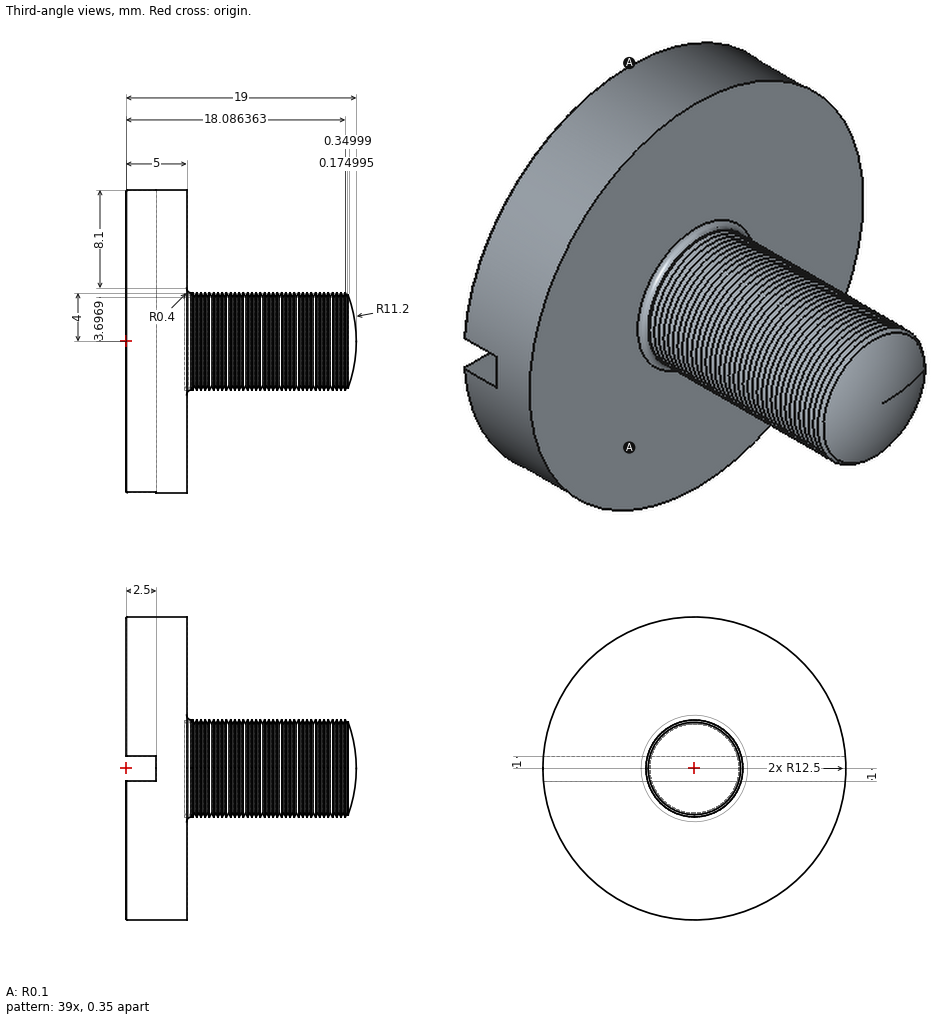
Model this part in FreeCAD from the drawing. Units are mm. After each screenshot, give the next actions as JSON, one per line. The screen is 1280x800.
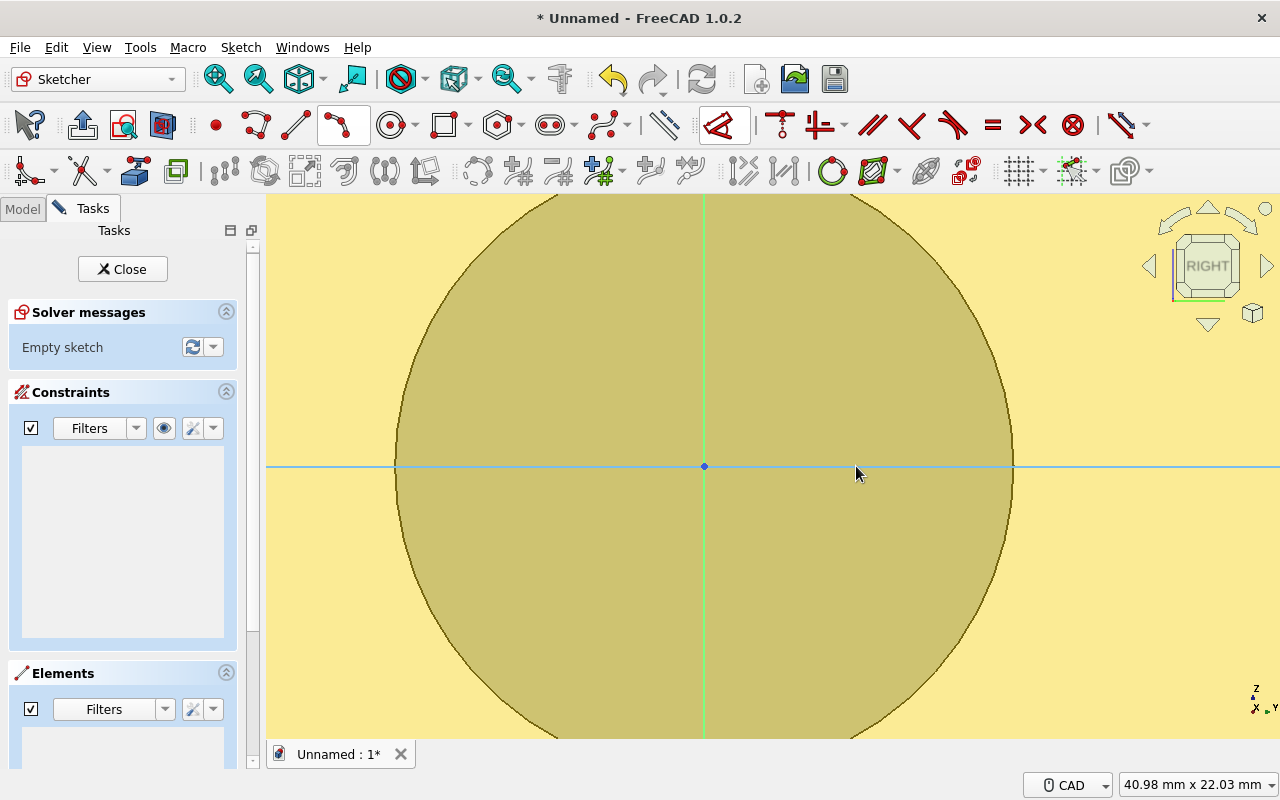
{"action": "left_click", "coordinate": [296, 126]}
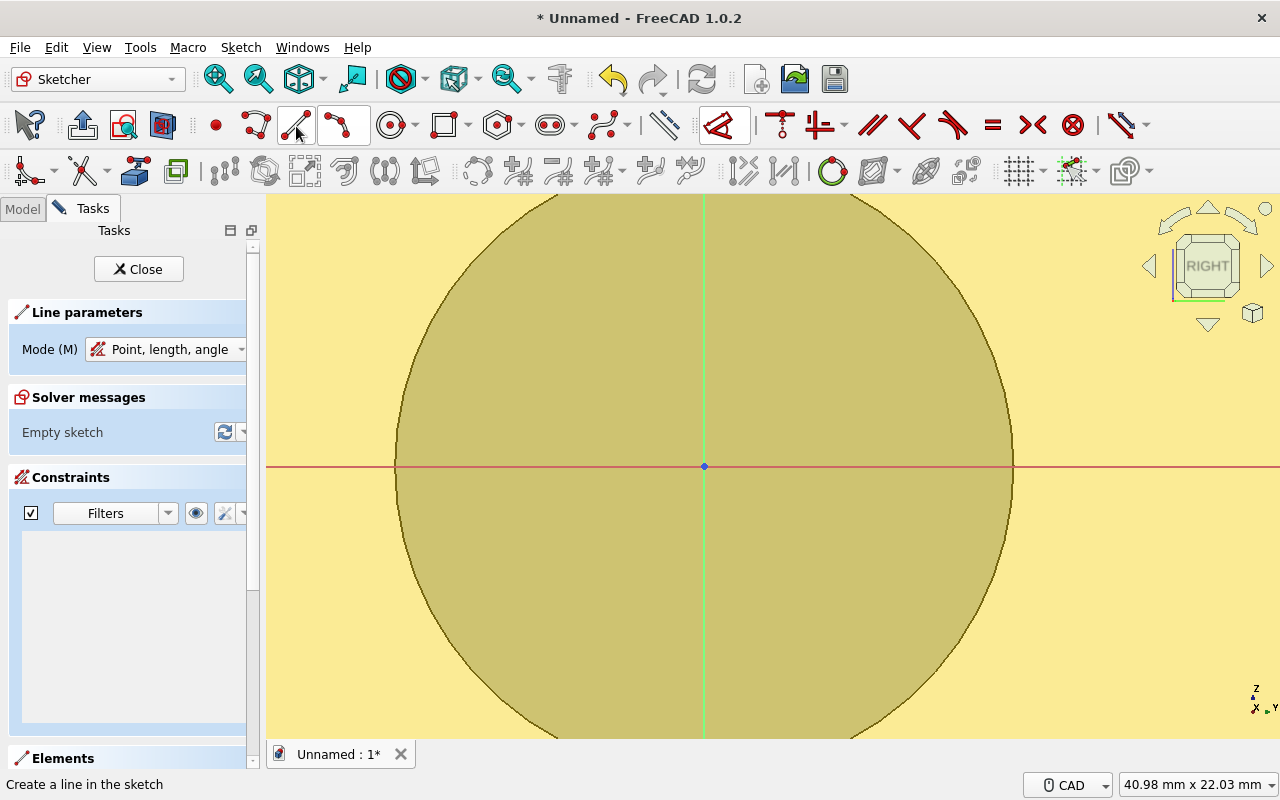
{"action": "left_click", "coordinate": [396, 442]}
{"action": "left_click", "coordinate": [1013, 442]}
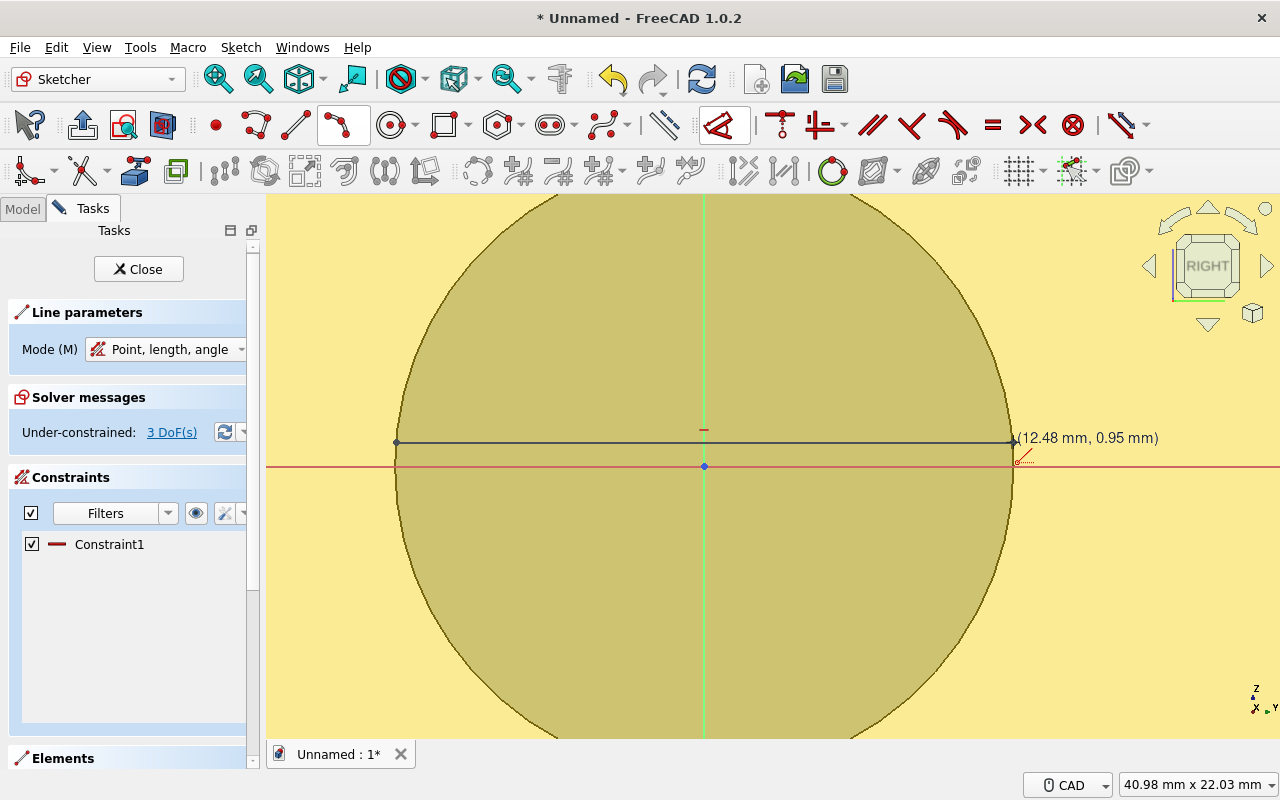
{"action": "left_click", "coordinate": [1013, 491]}
{"action": "left_click", "coordinate": [396, 491]}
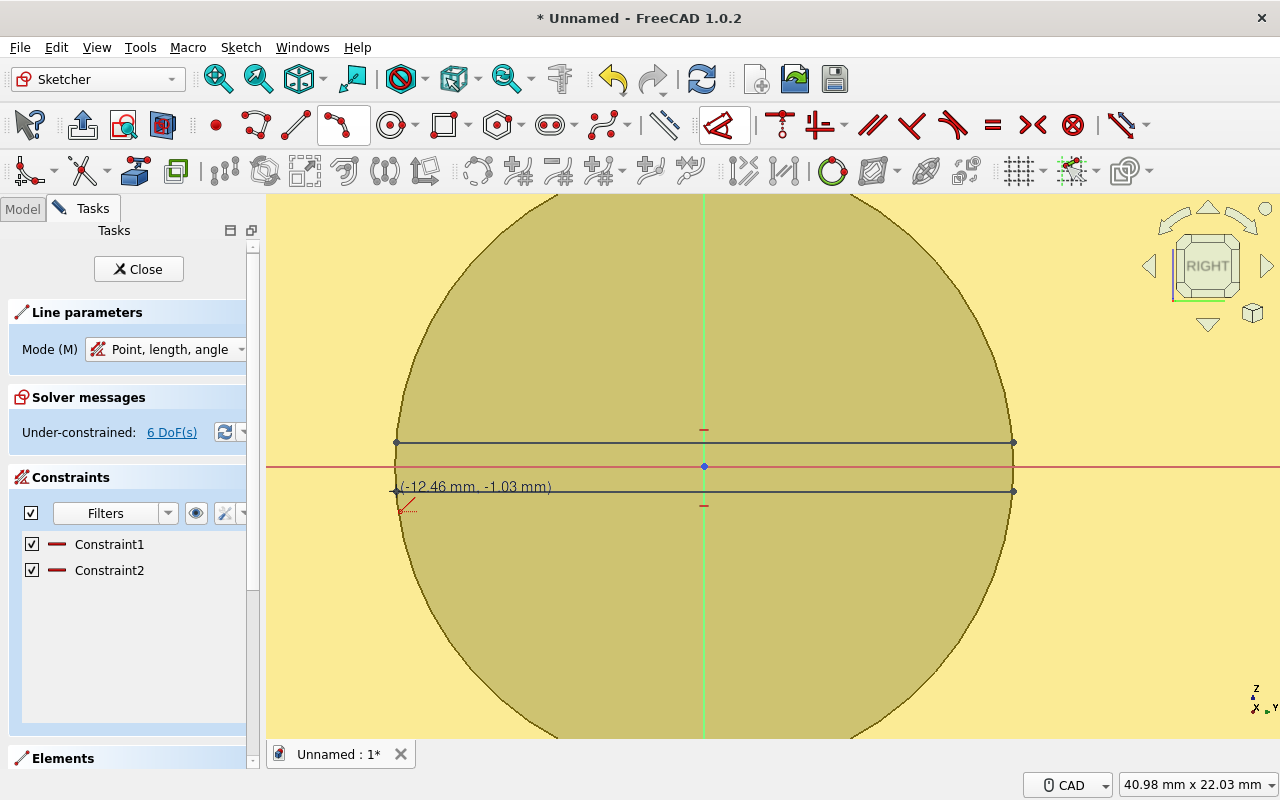
{"action": "left_click", "coordinate": [338, 126]}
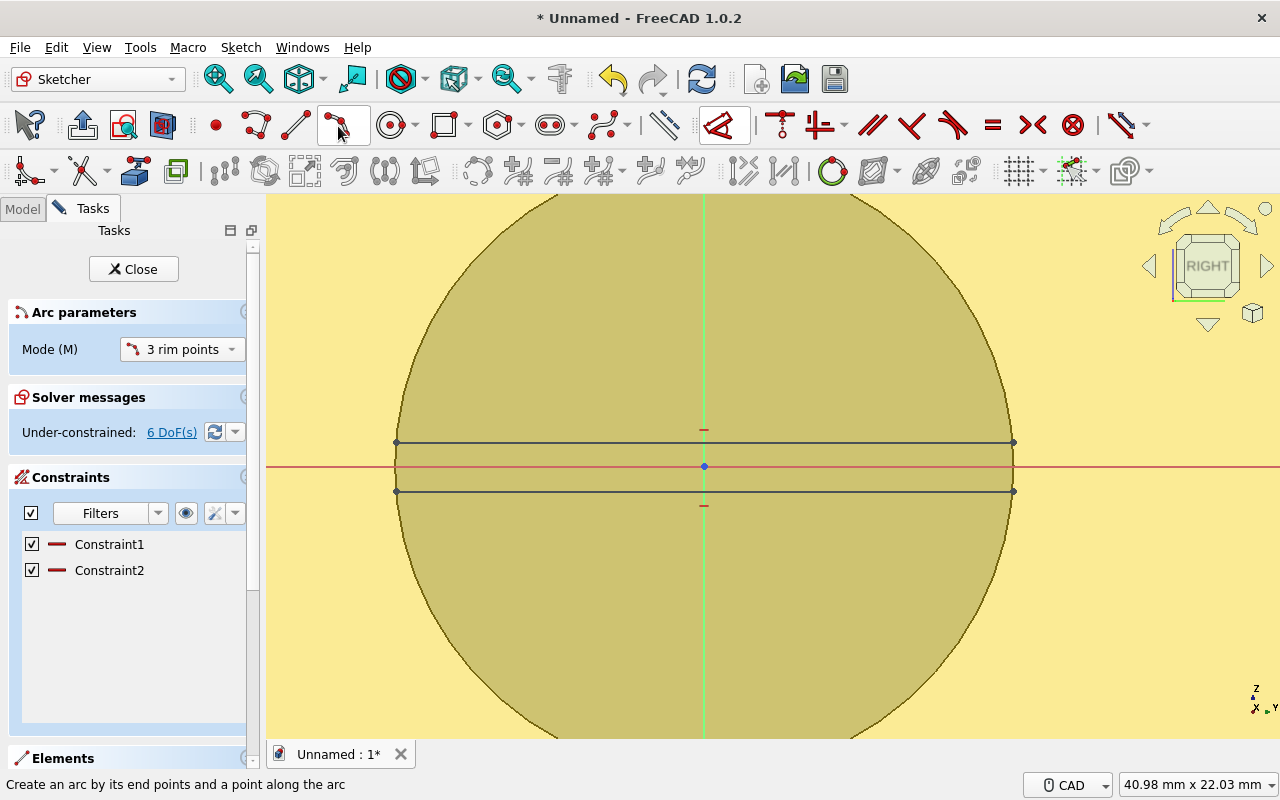
{"action": "left_click", "coordinate": [1013, 443]}
{"action": "left_click", "coordinate": [1013, 492]}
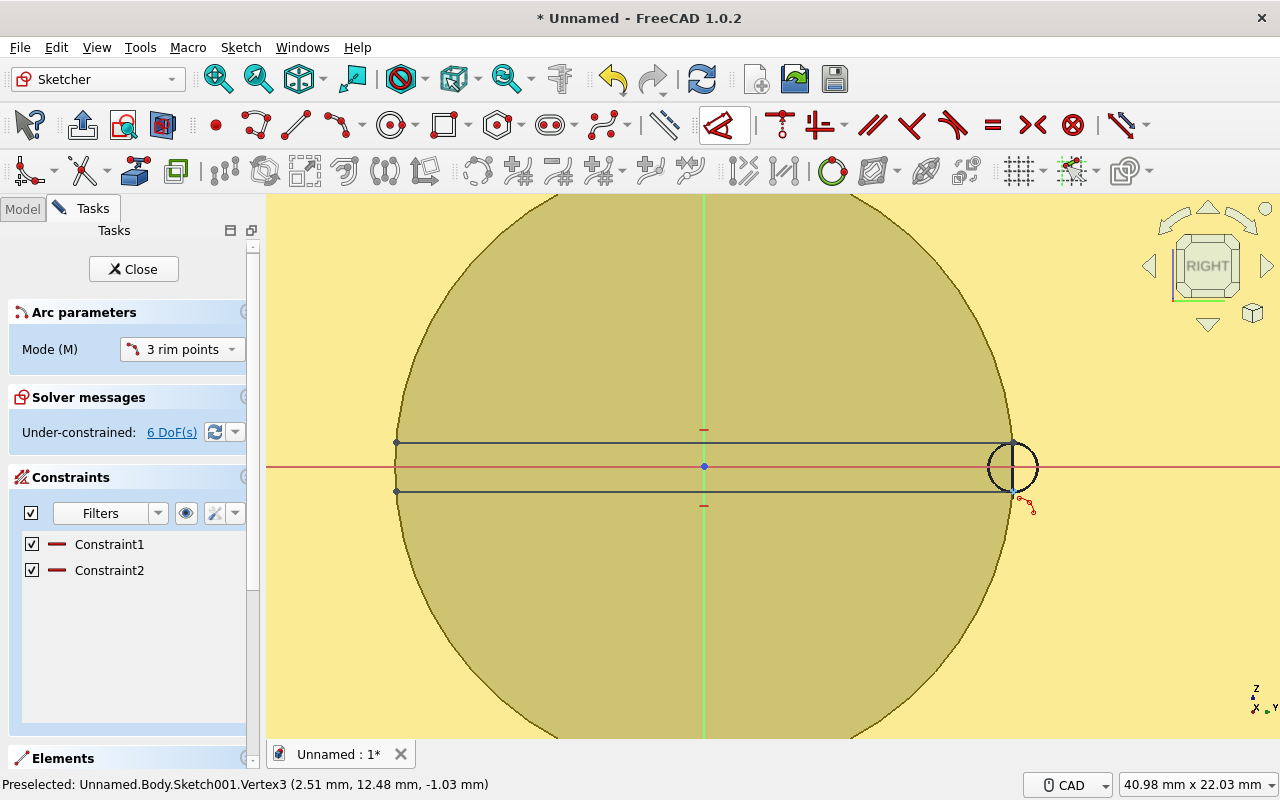
{"action": "scroll", "coordinate": [1014, 471], "scroll_direction": "up", "scroll_amount": 15}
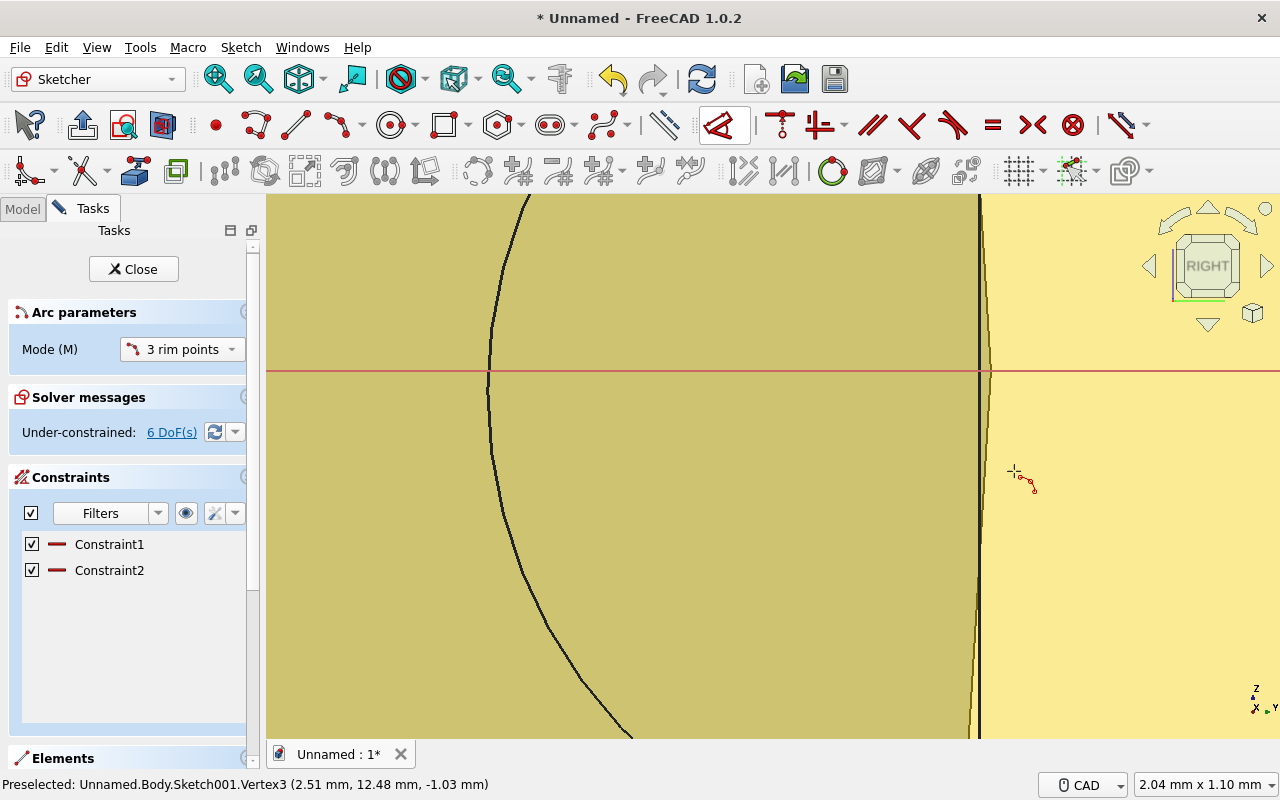
{"action": "left_click", "coordinate": [990, 470]}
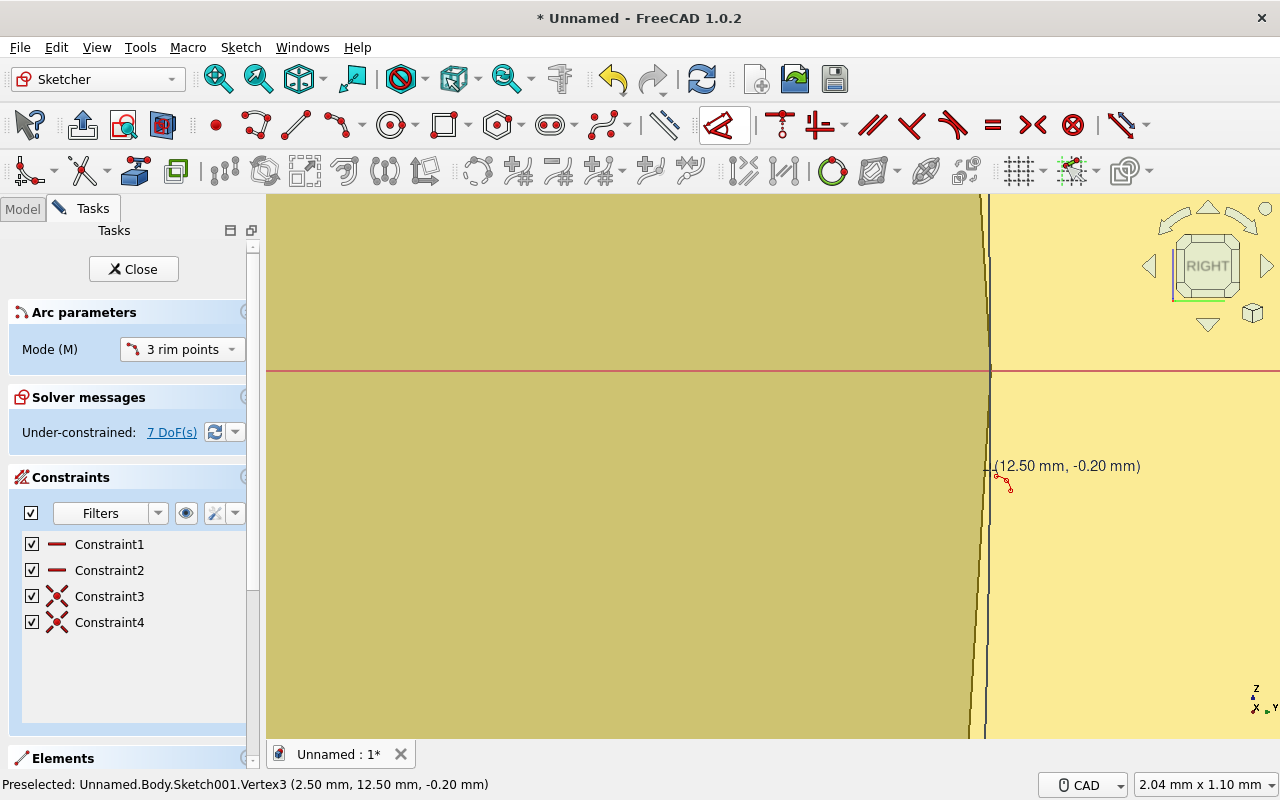
{"action": "scroll", "coordinate": [1015, 472], "scroll_direction": "down", "scroll_amount": 15}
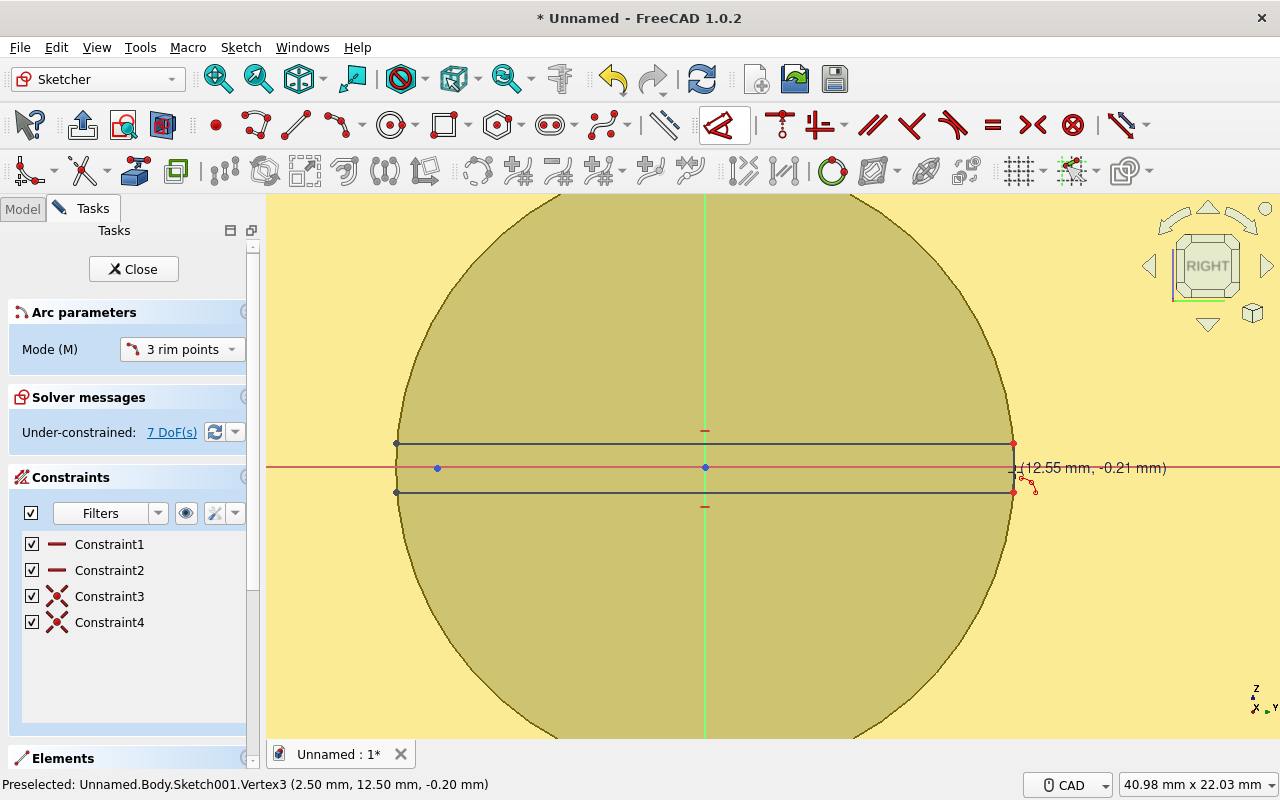
{"action": "left_click", "coordinate": [397, 493]}
{"action": "left_click", "coordinate": [397, 444]}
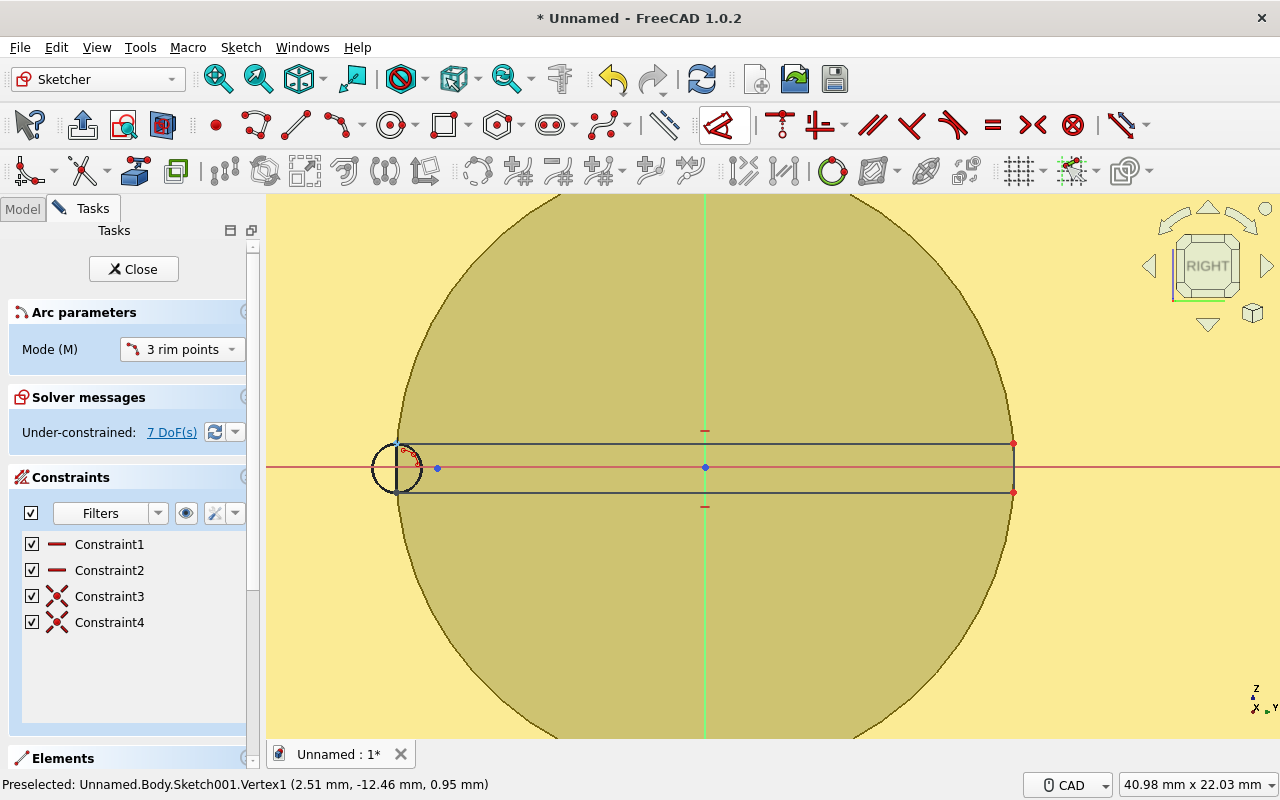
{"action": "scroll", "coordinate": [396, 472], "scroll_direction": "up", "scroll_amount": 15}